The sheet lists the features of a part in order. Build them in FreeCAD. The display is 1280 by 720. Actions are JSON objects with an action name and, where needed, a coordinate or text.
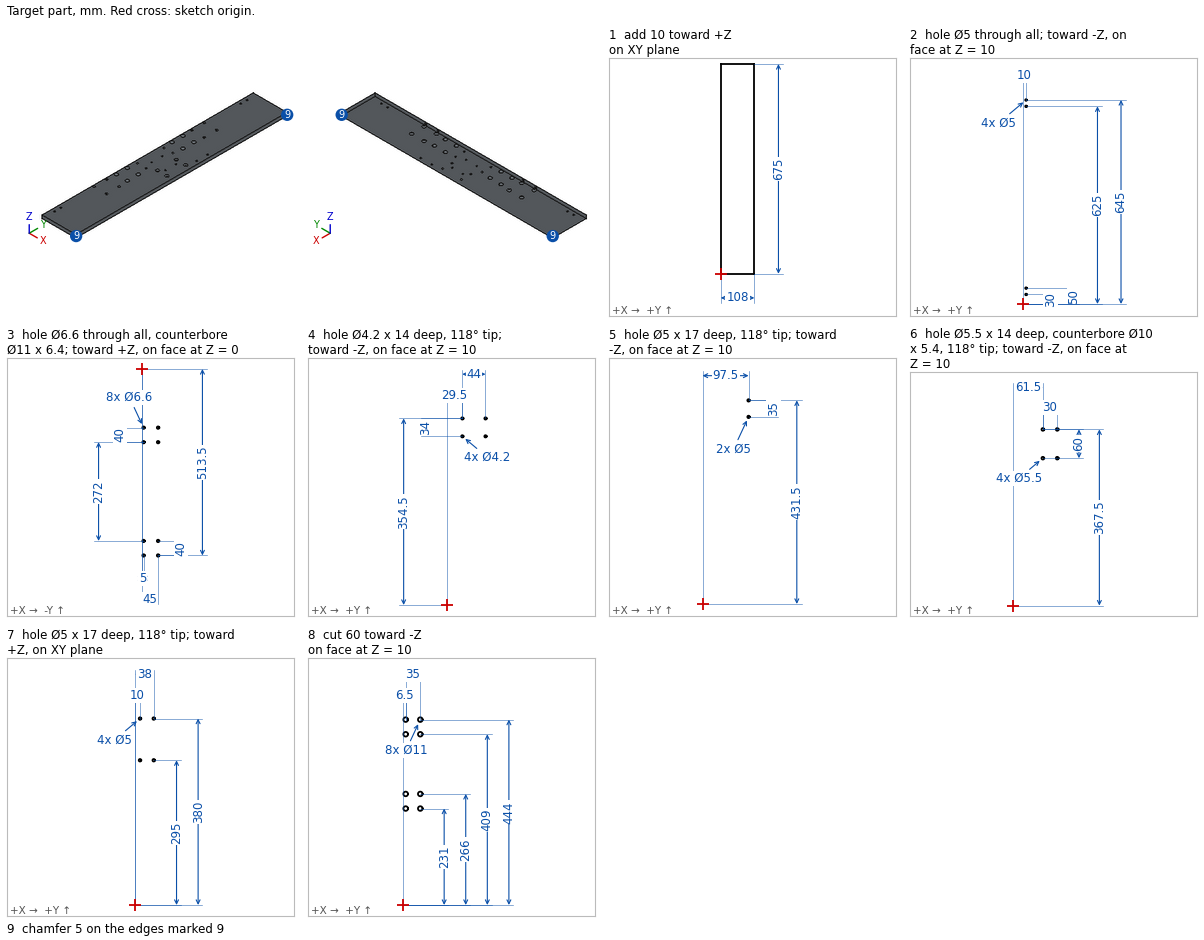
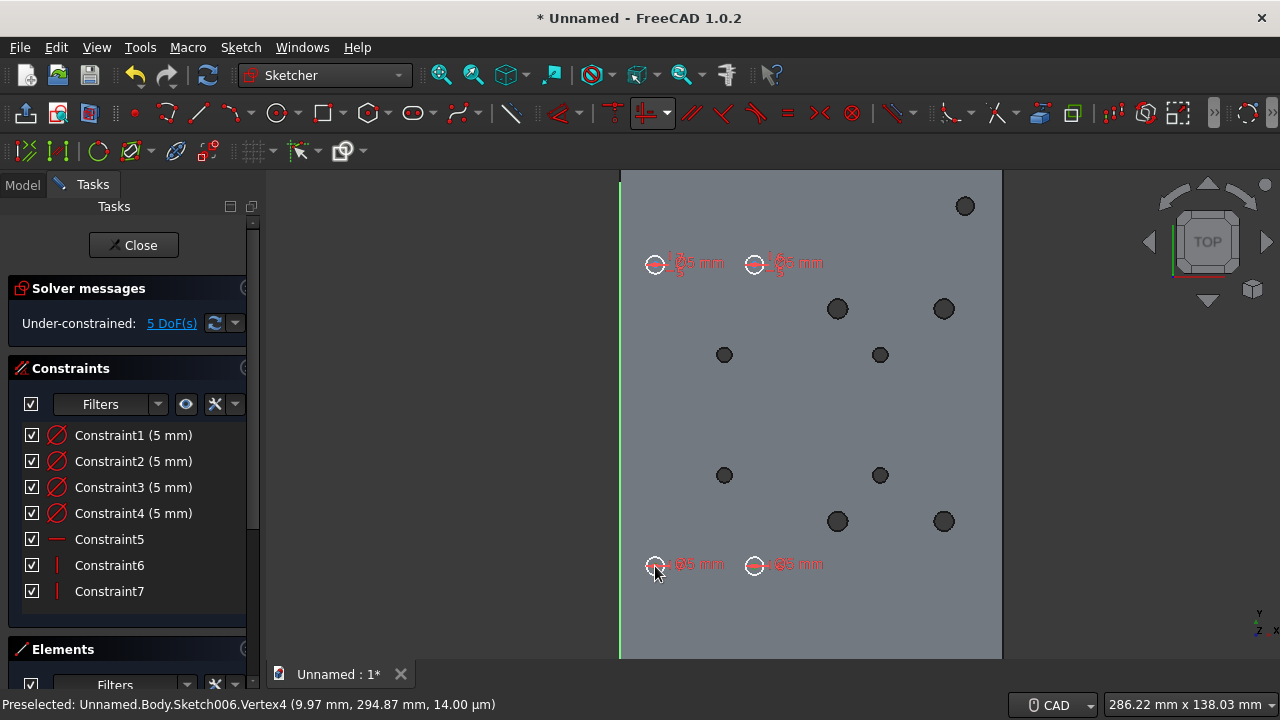
{"action": "key", "text": "h"}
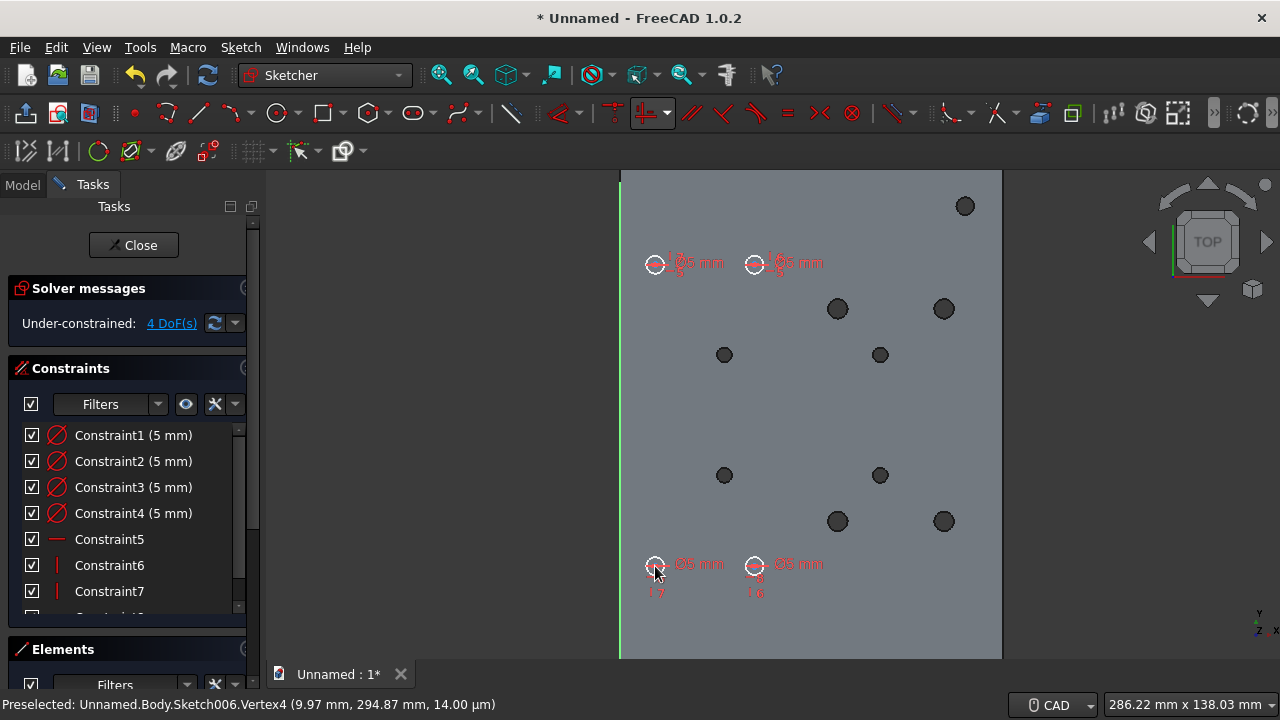
{"action": "left_click", "coordinate": [558, 114]}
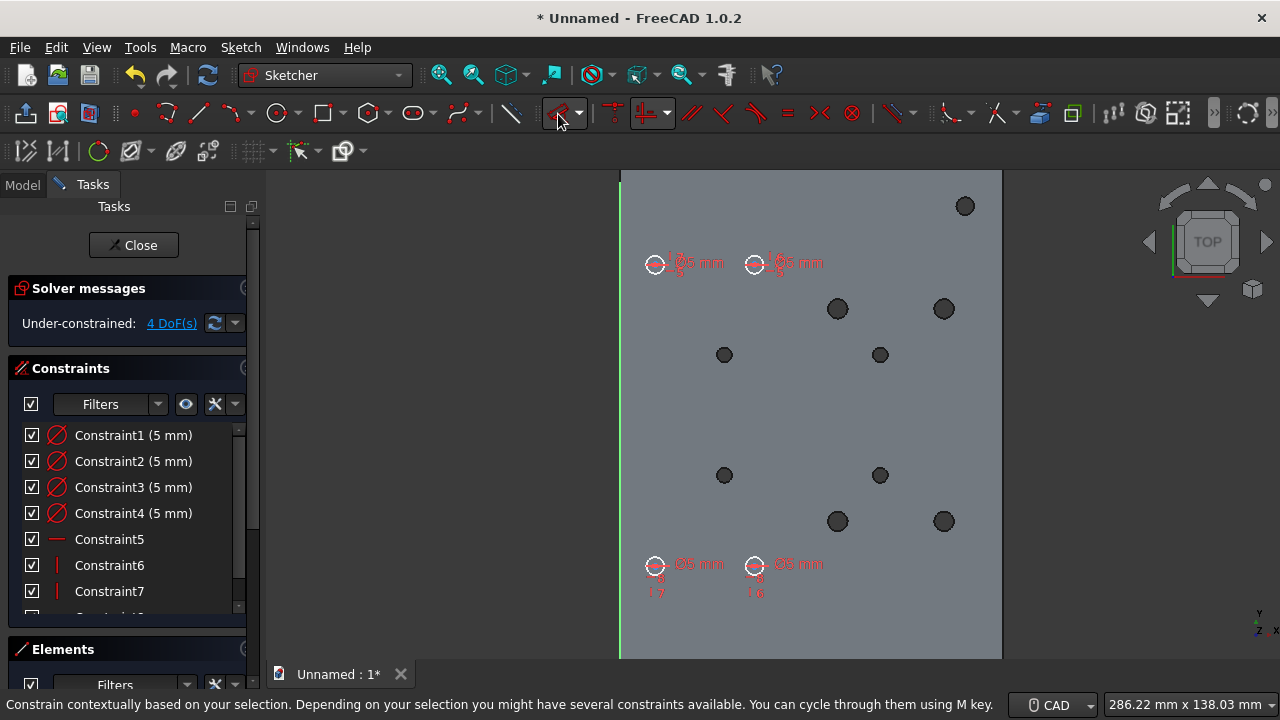
{"action": "left_click", "coordinate": [755, 265]}
{"action": "left_click", "coordinate": [687, 231]}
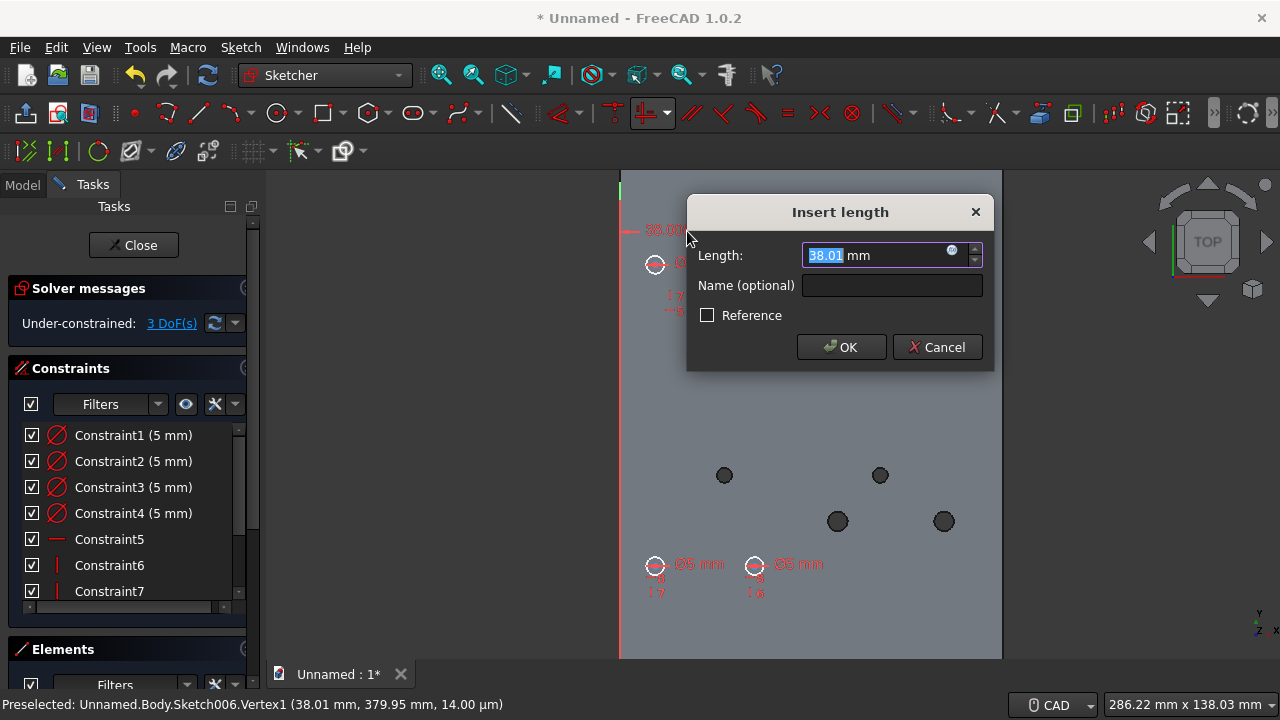
{"action": "type", "text": "38"}
{"action": "key", "text": "Return"}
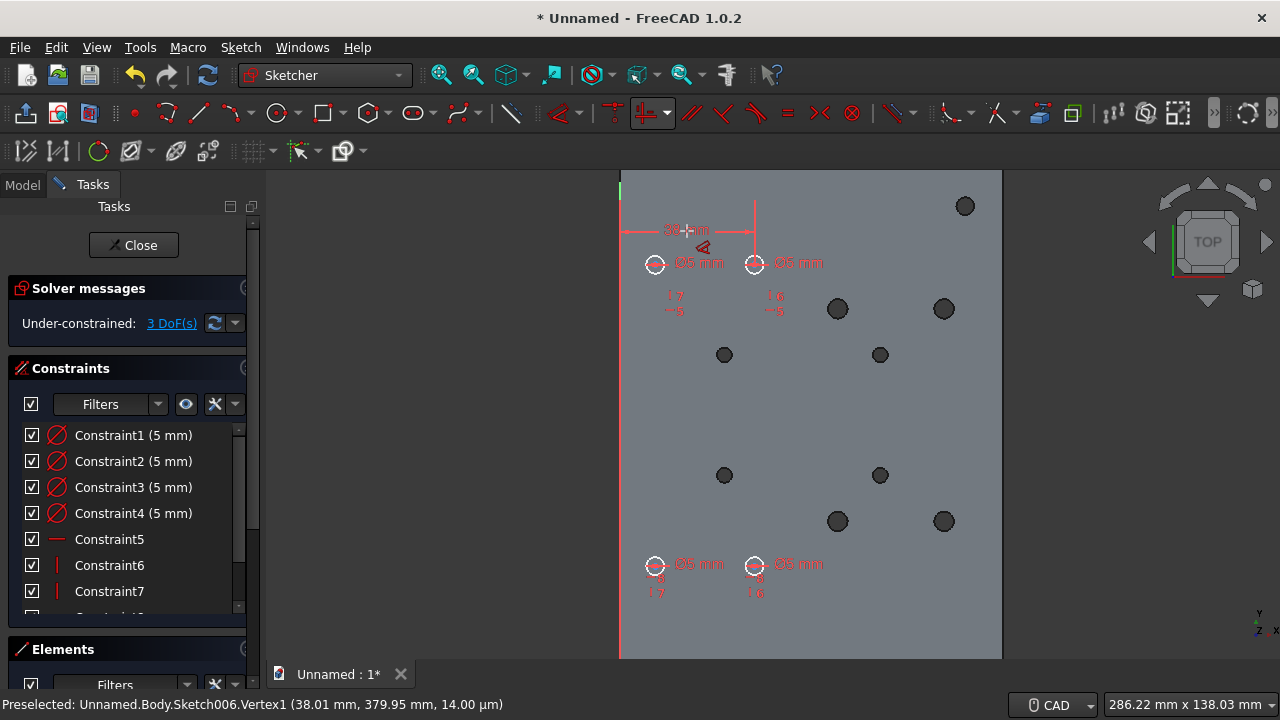
{"action": "left_click", "coordinate": [655, 265]}
{"action": "left_click", "coordinate": [638, 207]}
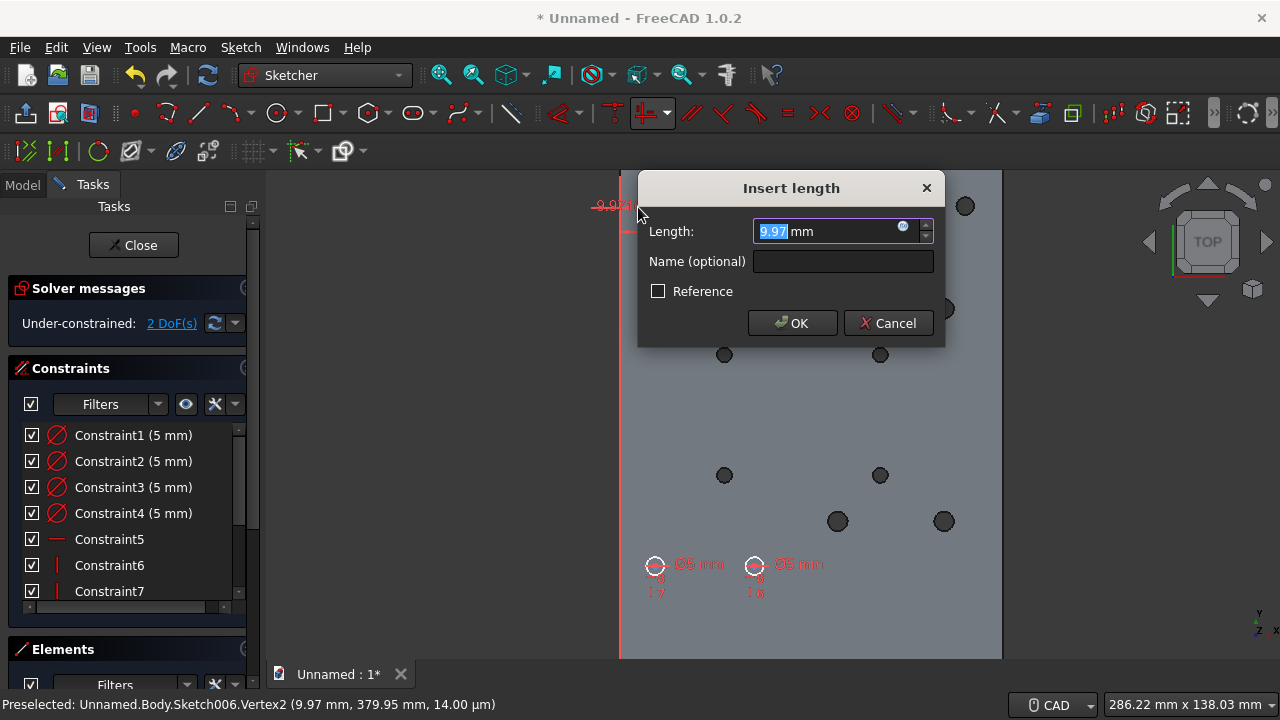
{"action": "type", "text": "10"}
{"action": "key", "text": "Return"}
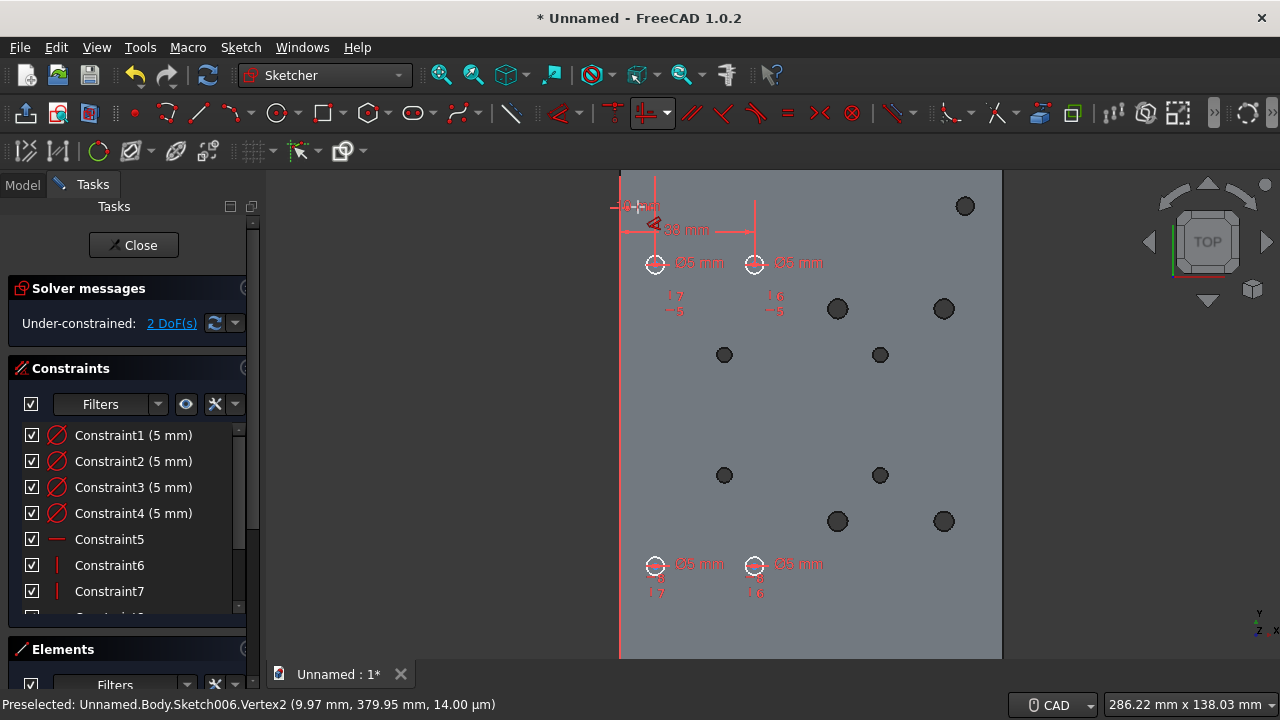
{"action": "left_click", "coordinate": [755, 265]}
{"action": "left_click", "coordinate": [586, 448]}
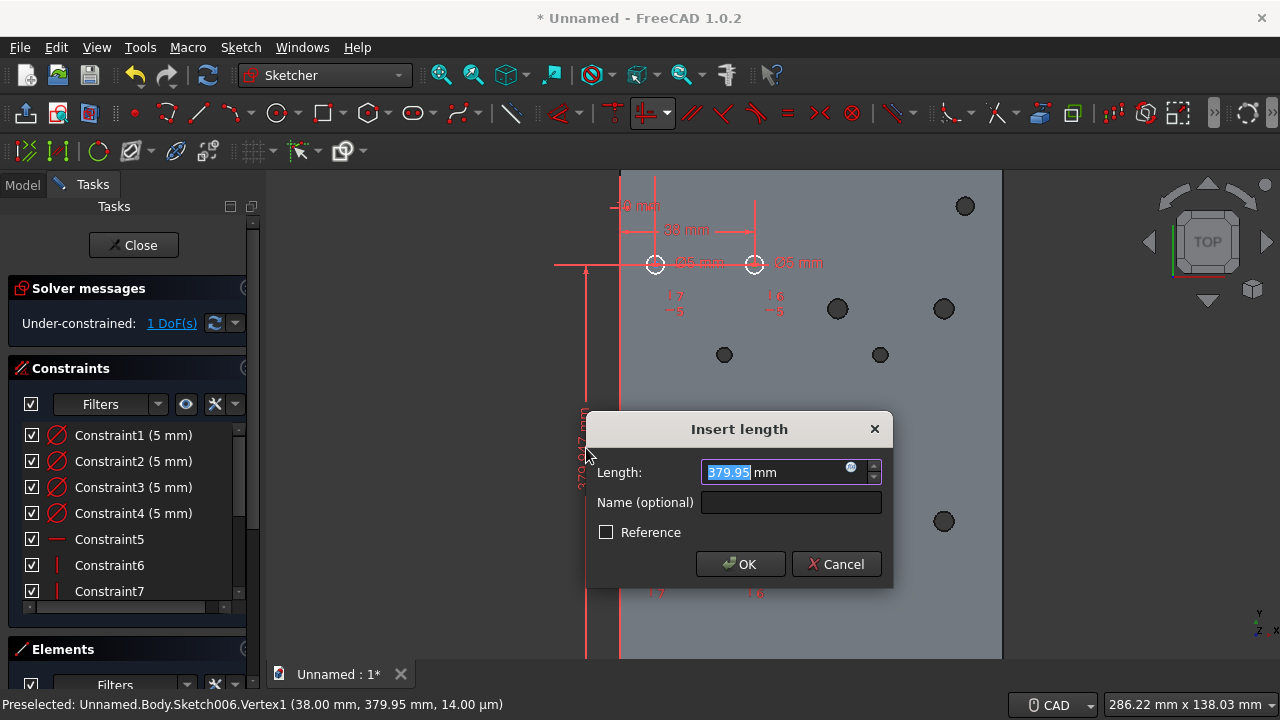
{"action": "type", "text": "380"}
{"action": "key", "text": "Return"}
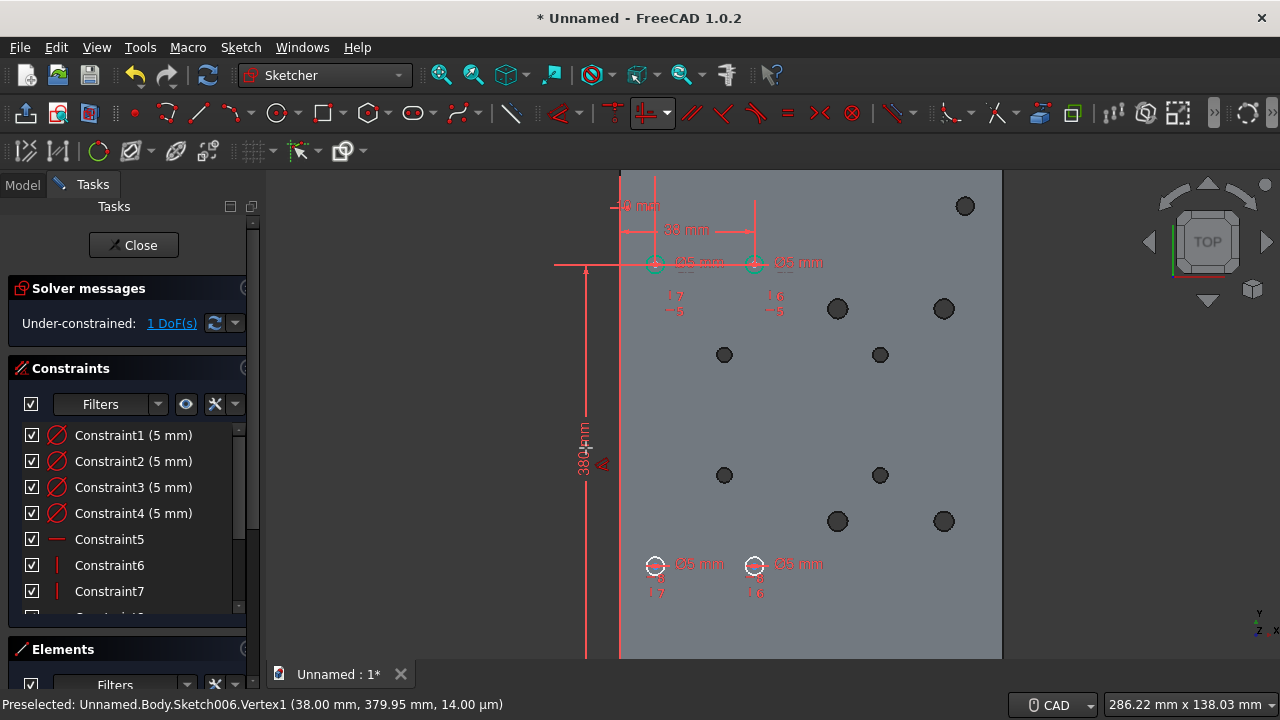
{"action": "left_click", "coordinate": [755, 566]}
{"action": "left_click", "coordinate": [586, 599]}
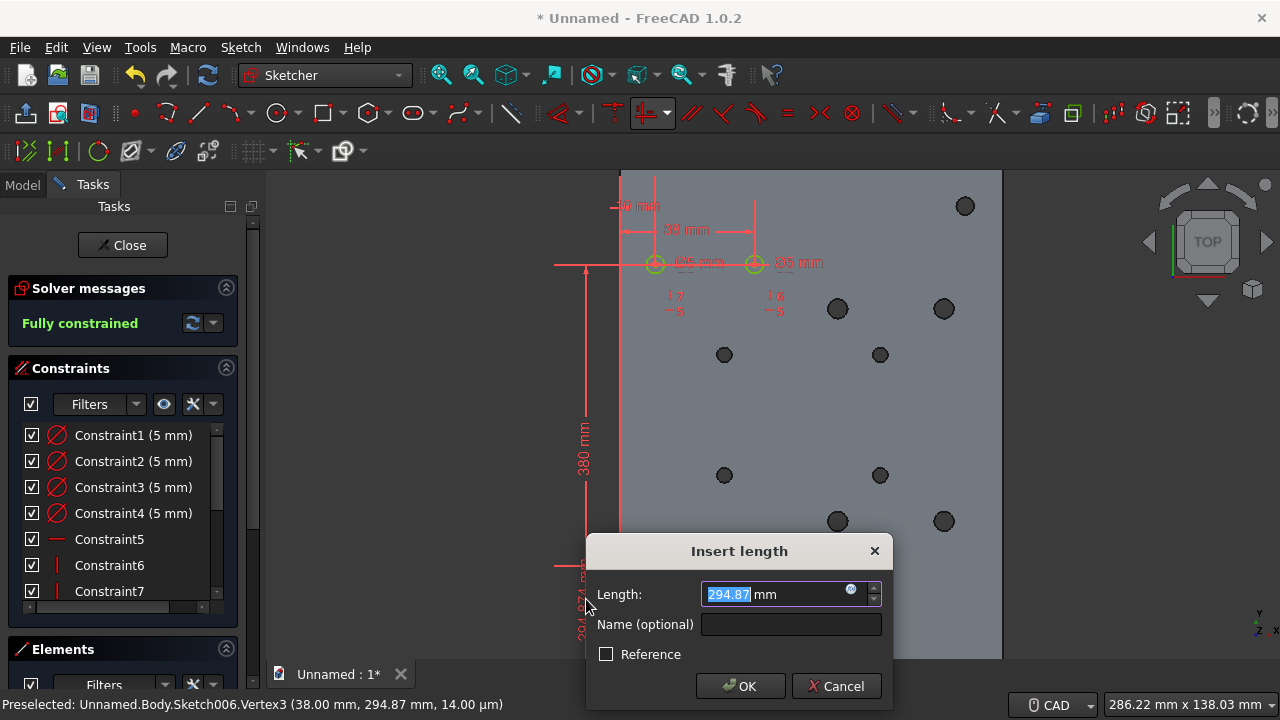
{"action": "type", "text": "295"}
{"action": "key", "text": "Return"}
{"action": "key", "text": "Escape"}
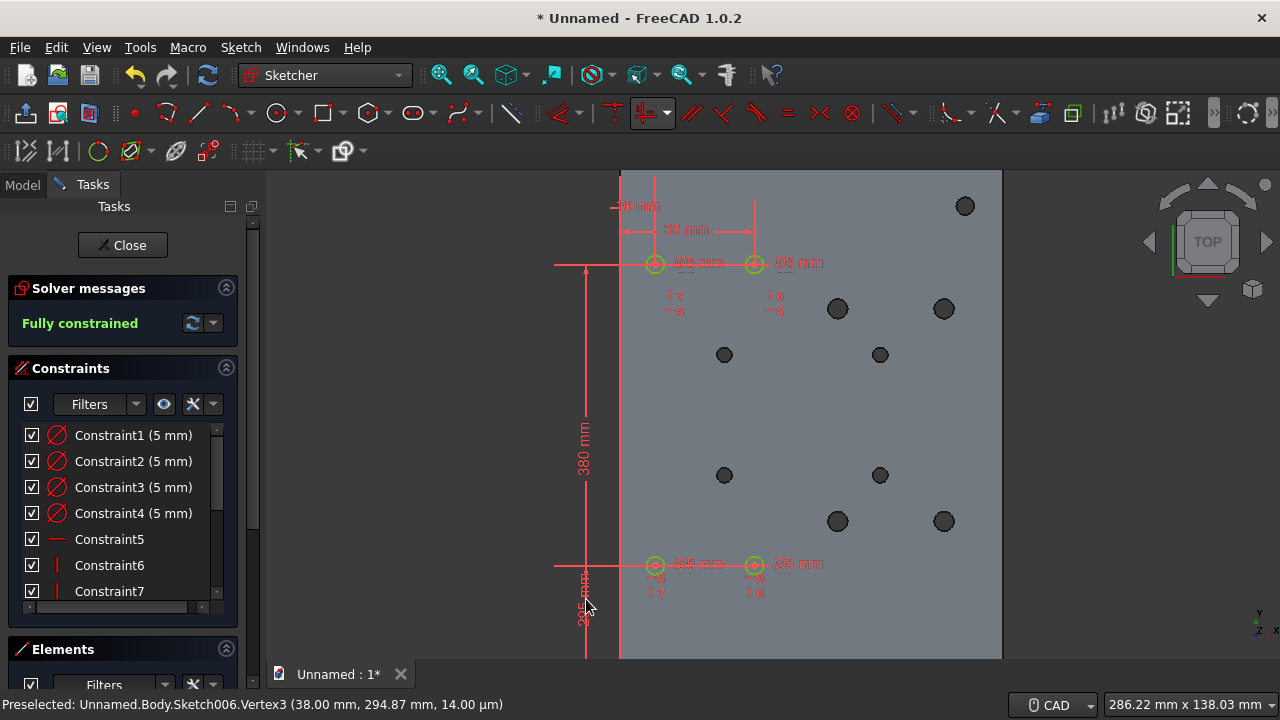
{"action": "left_click", "coordinate": [123, 245]}